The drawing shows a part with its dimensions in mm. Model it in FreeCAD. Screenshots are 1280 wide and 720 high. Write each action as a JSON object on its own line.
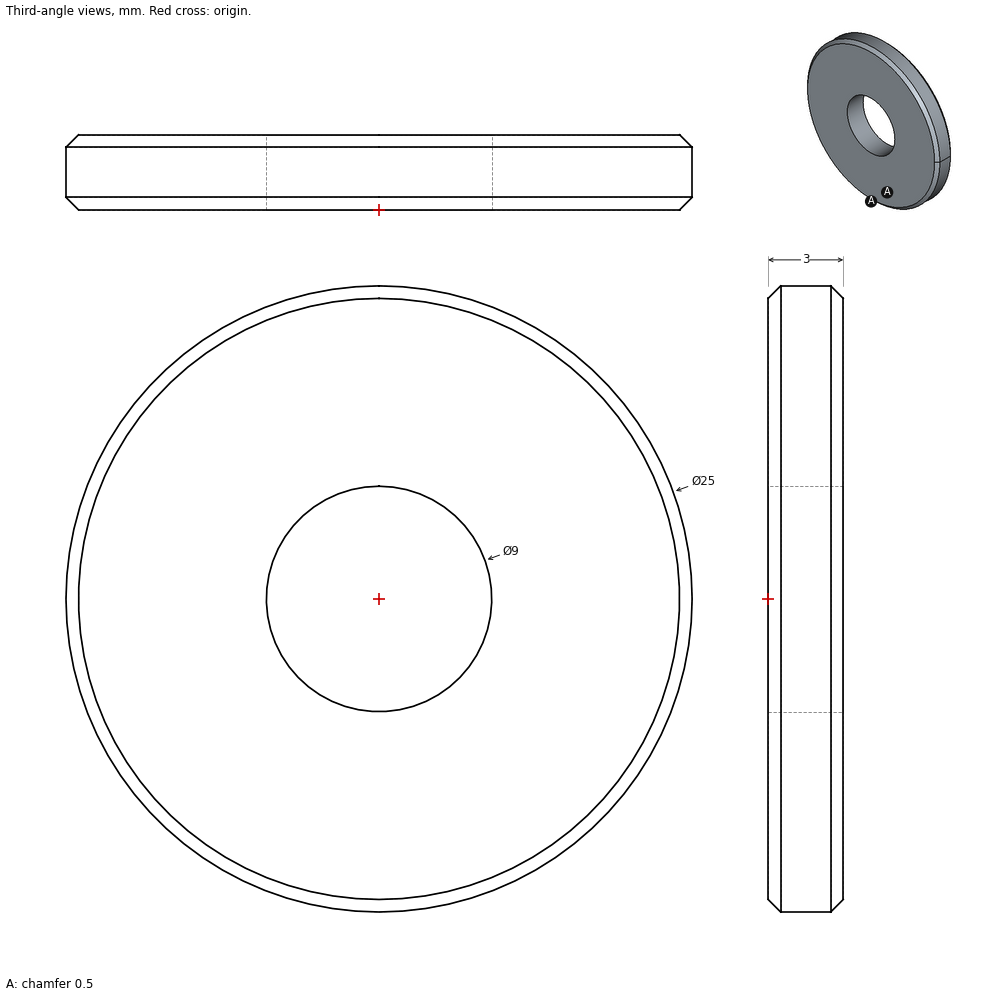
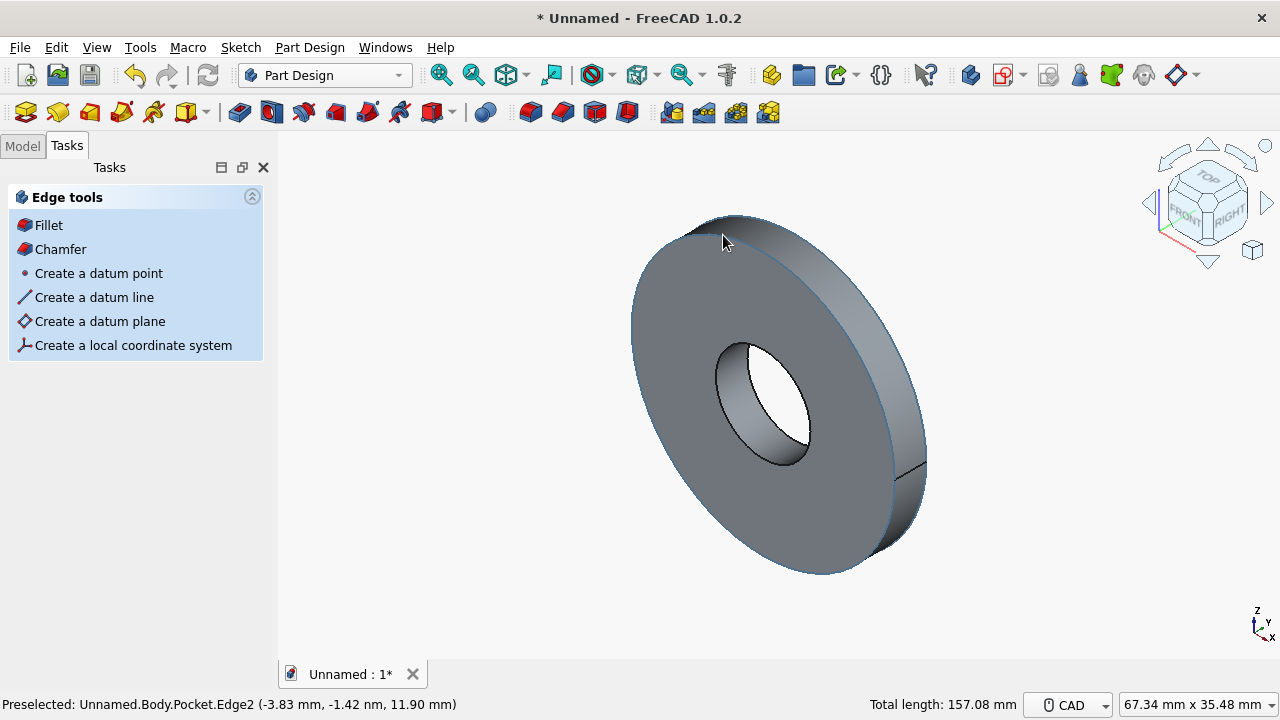
{"action": "left_click", "coordinate": [564, 112]}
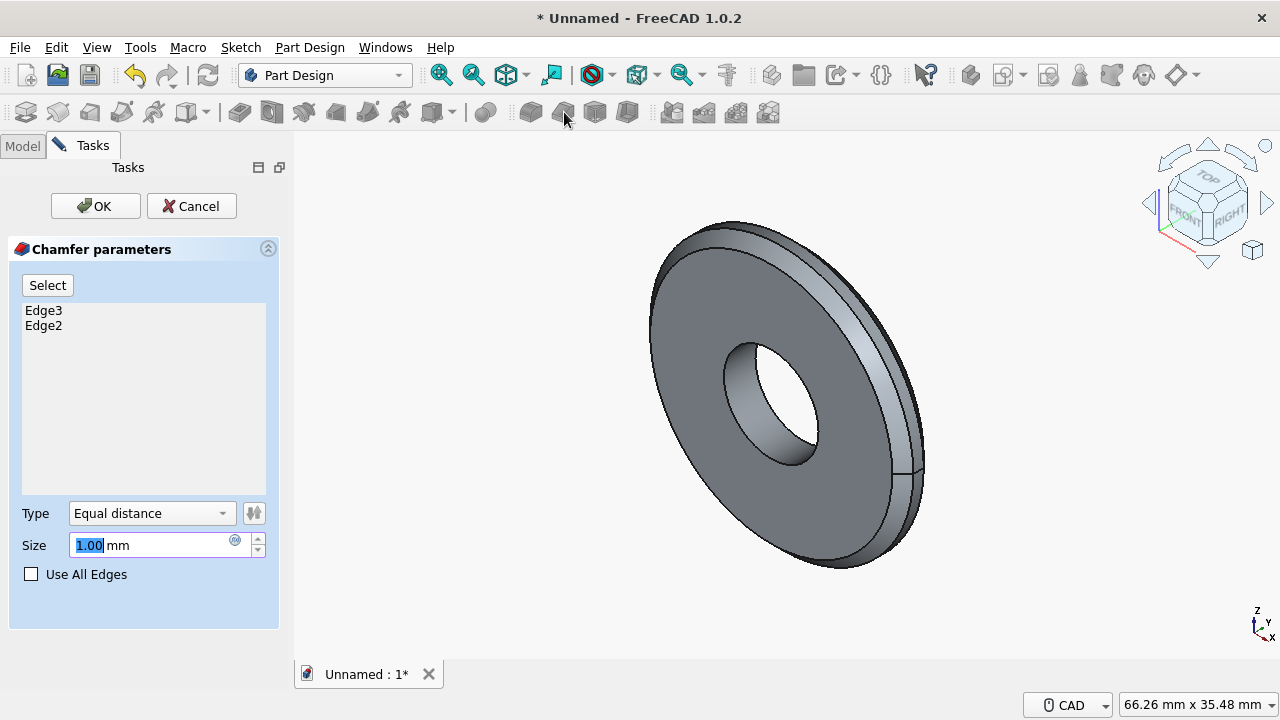
{"action": "type", "text": "0.5"}
{"action": "key", "text": "Tab"}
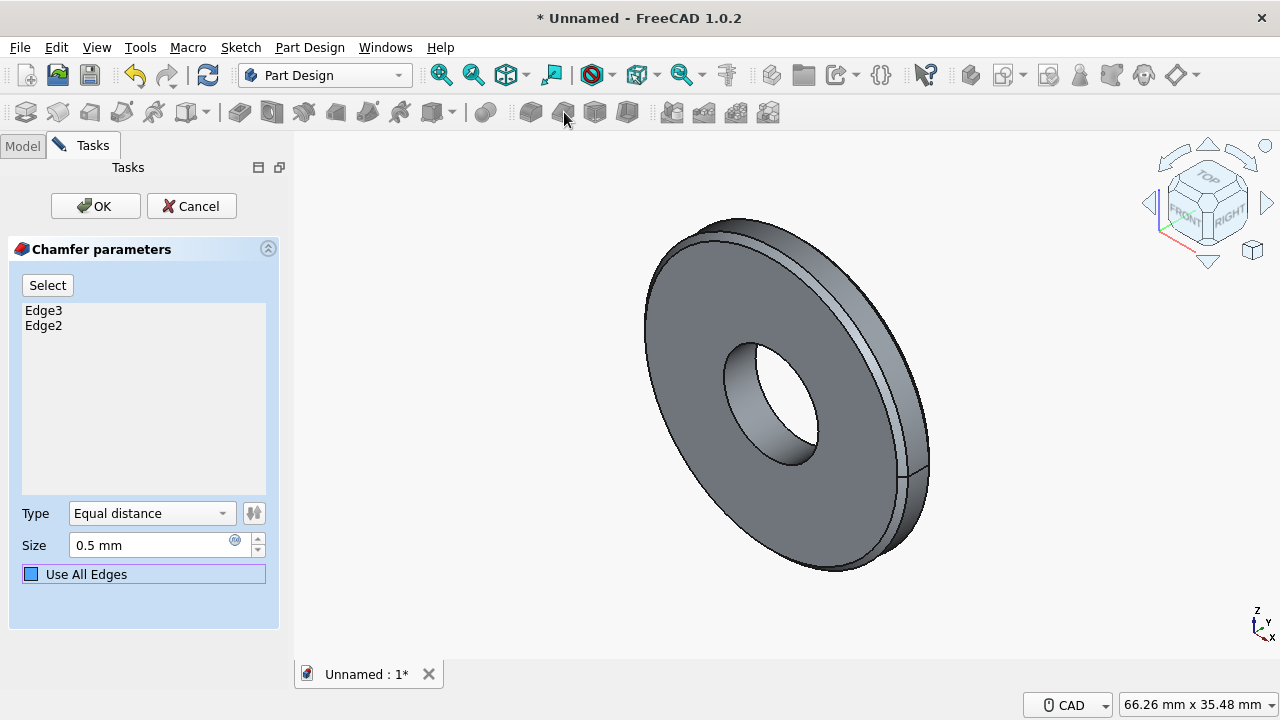
{"action": "left_click", "coordinate": [96, 206]}